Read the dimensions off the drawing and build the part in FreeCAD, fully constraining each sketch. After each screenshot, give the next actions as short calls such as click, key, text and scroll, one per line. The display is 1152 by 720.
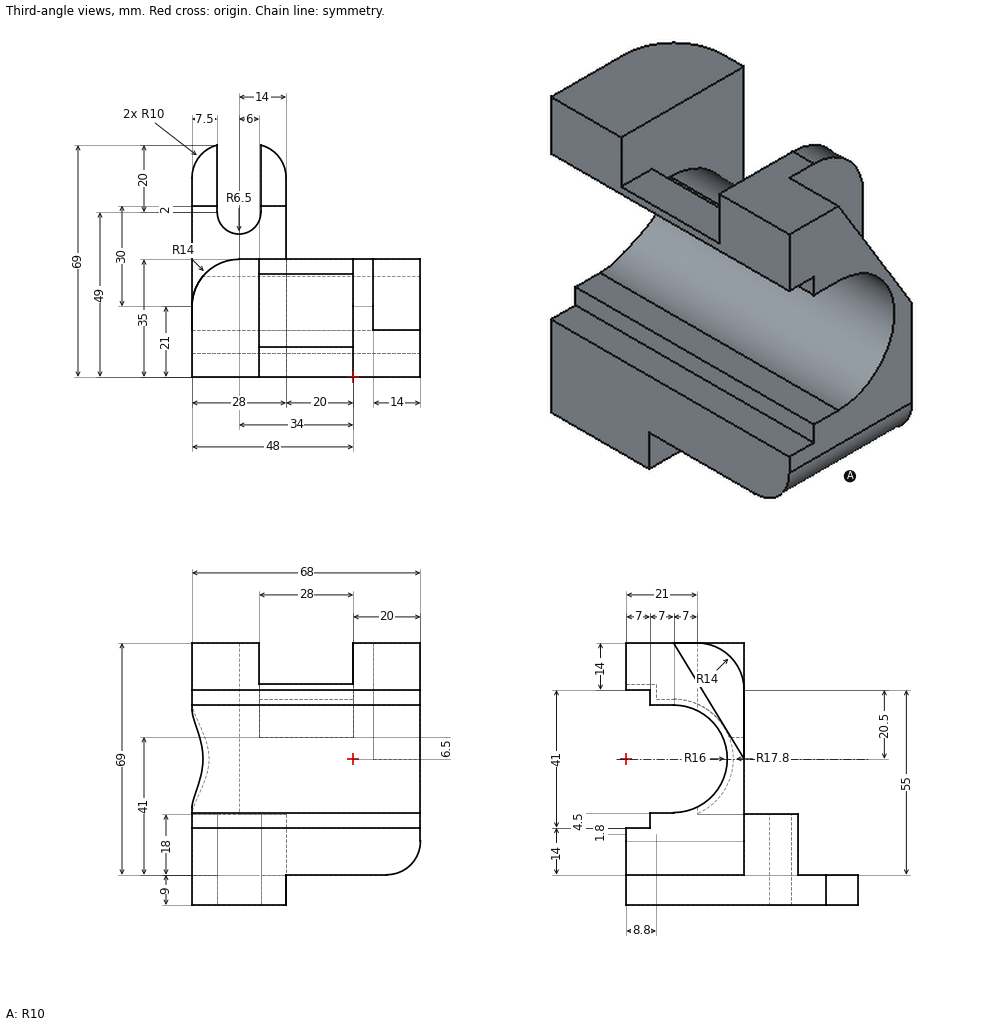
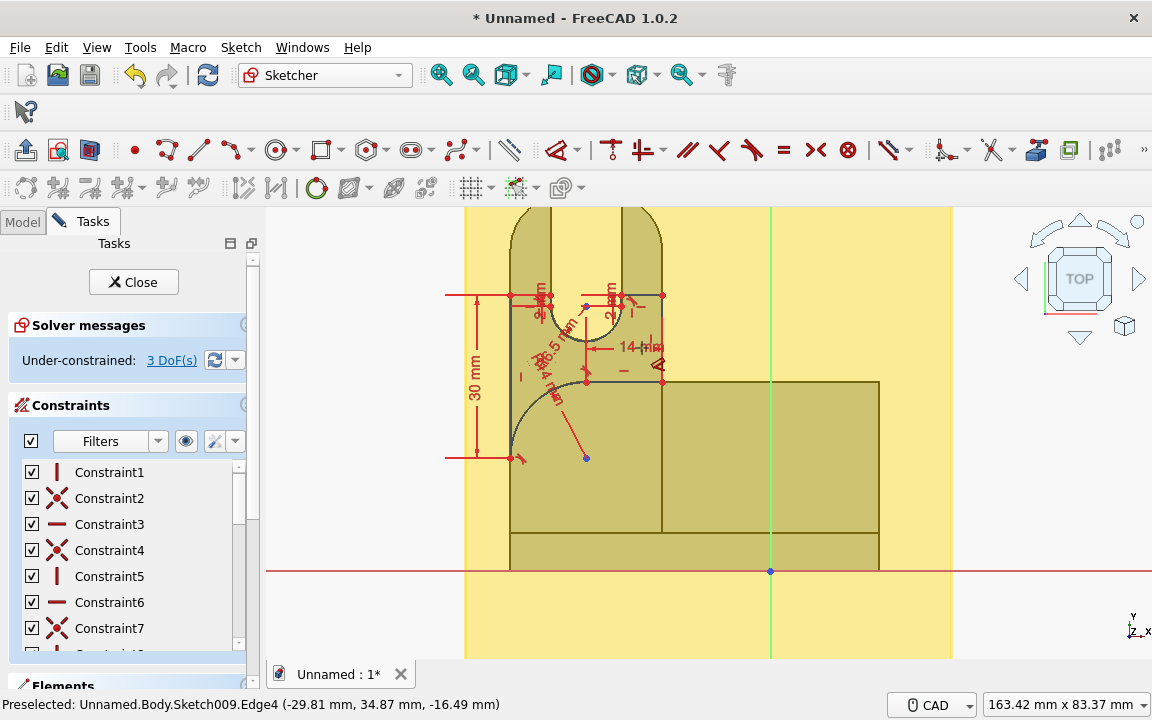
click(539, 295)
click(531, 261)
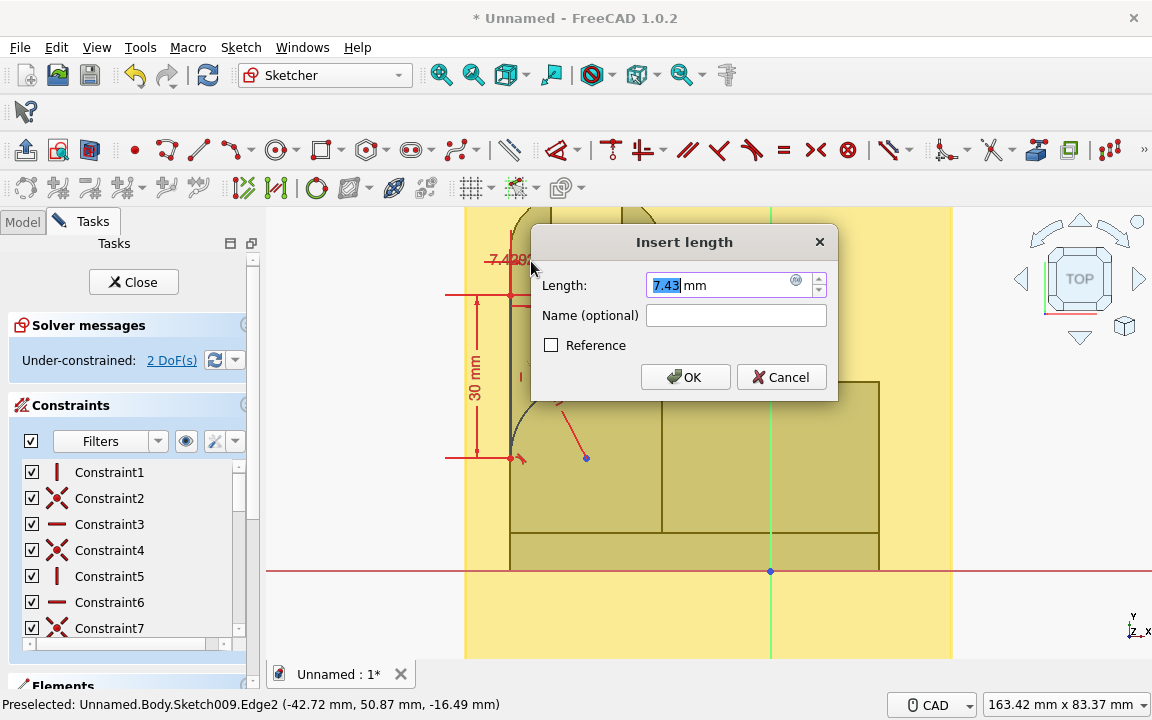
text(7.5)
key(Return)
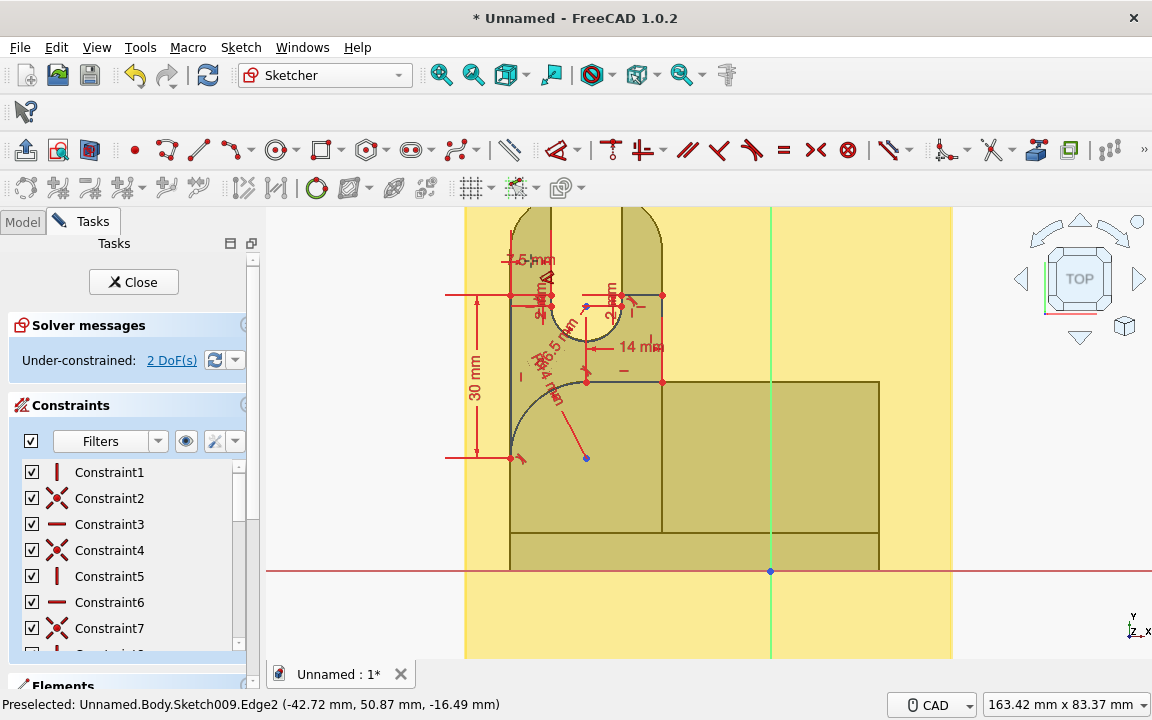
click(551, 306)
click(805, 439)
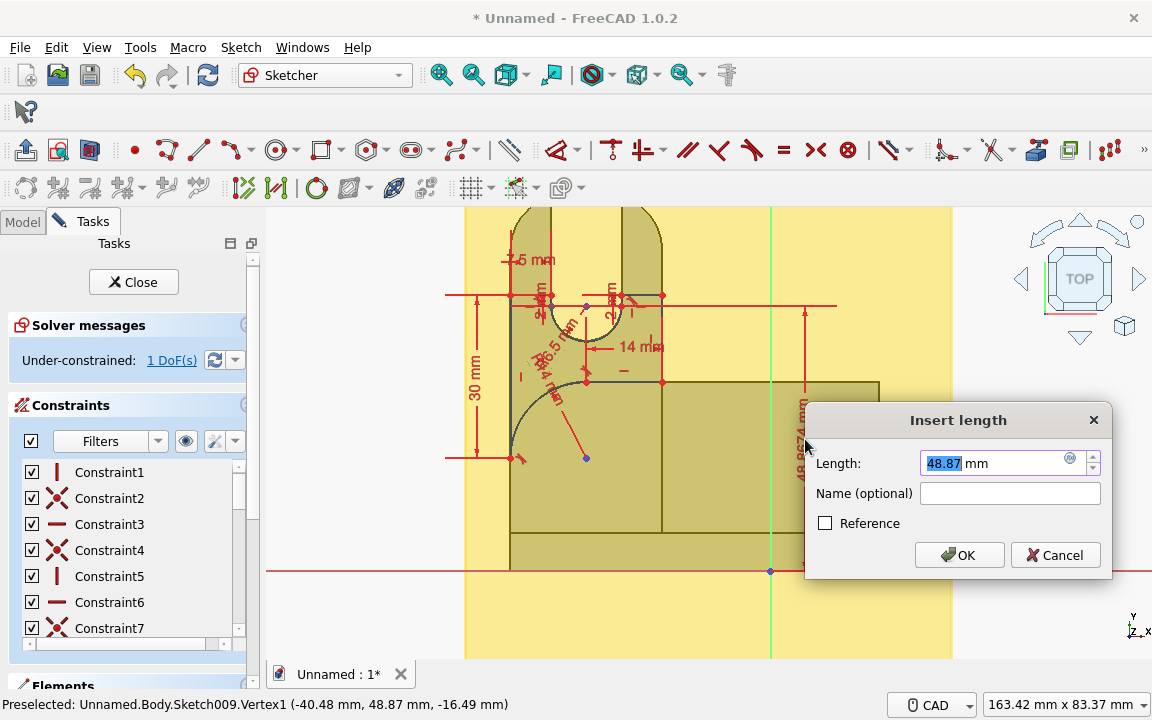
text(49)
key(Return)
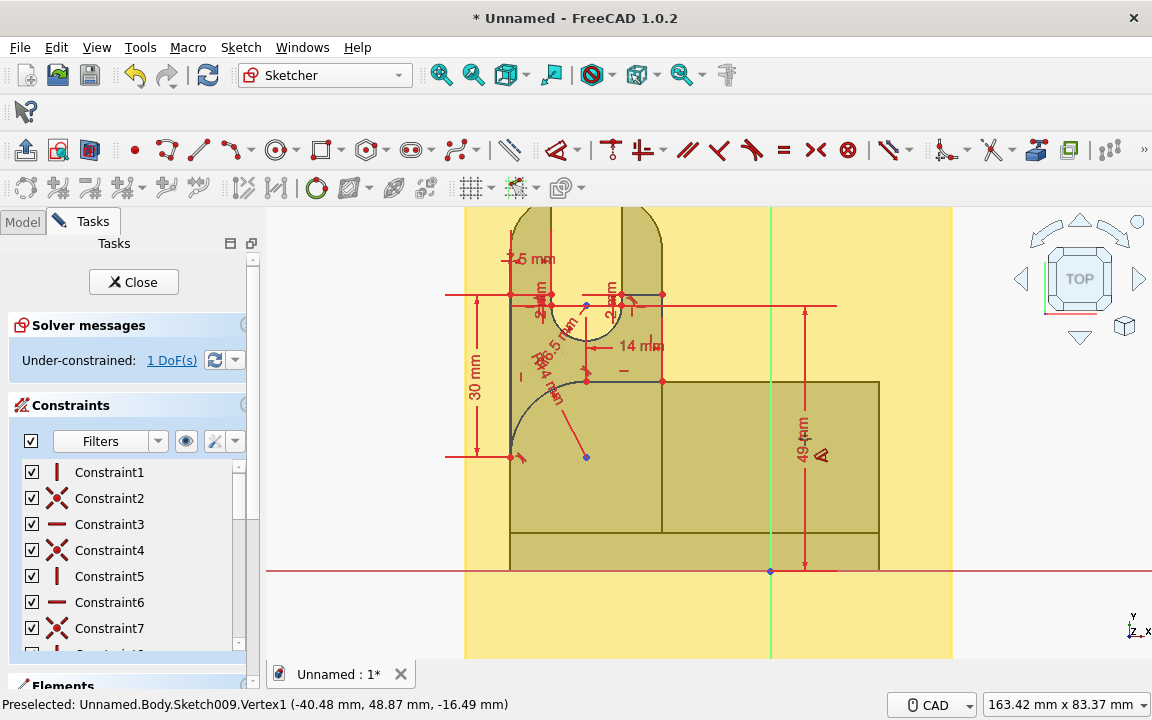
click(511, 295)
click(641, 605)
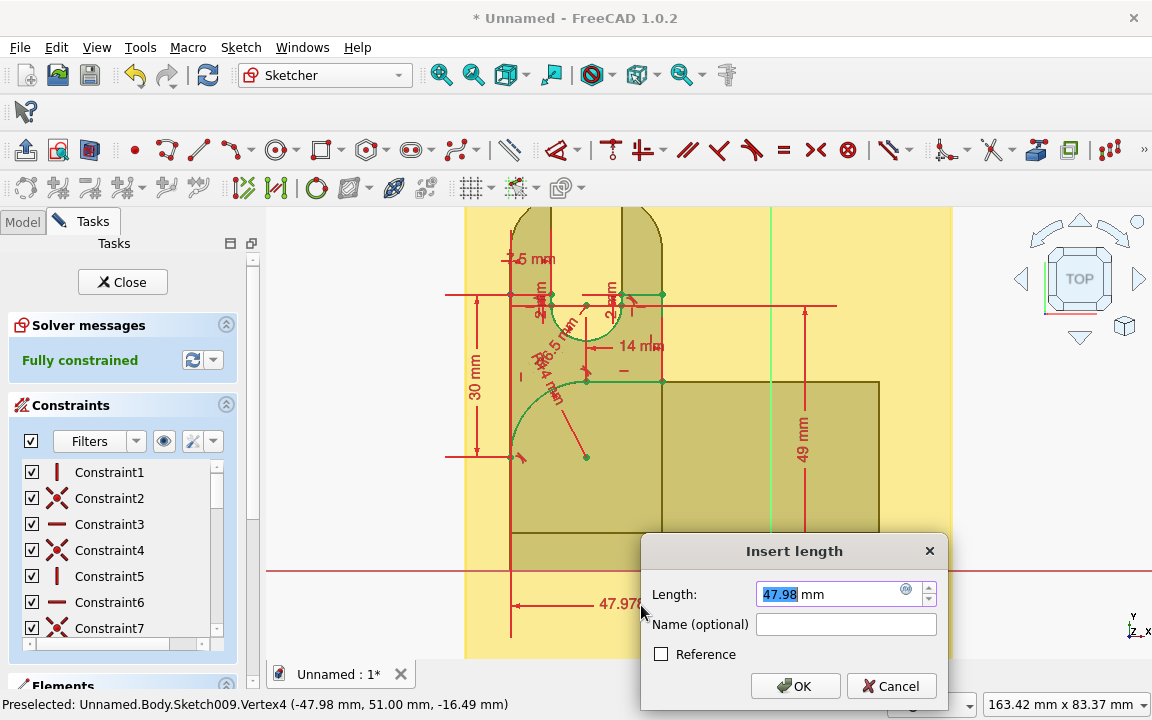
text(48)
key(Return)
key(Escape)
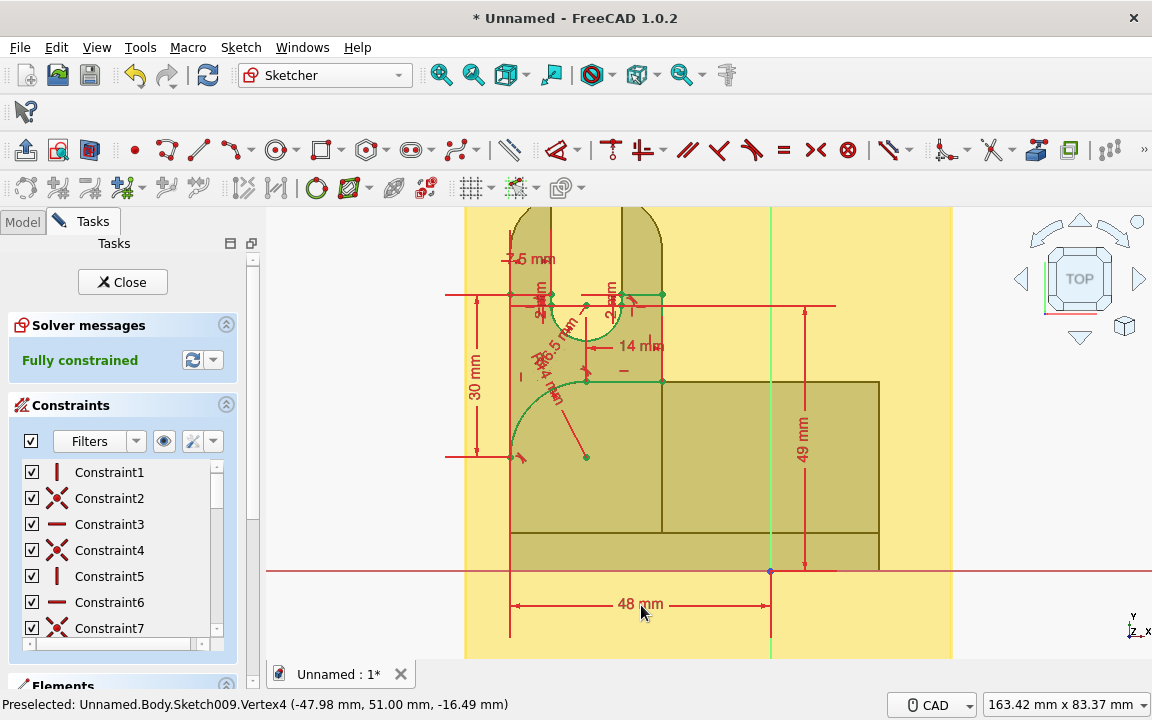
click(123, 282)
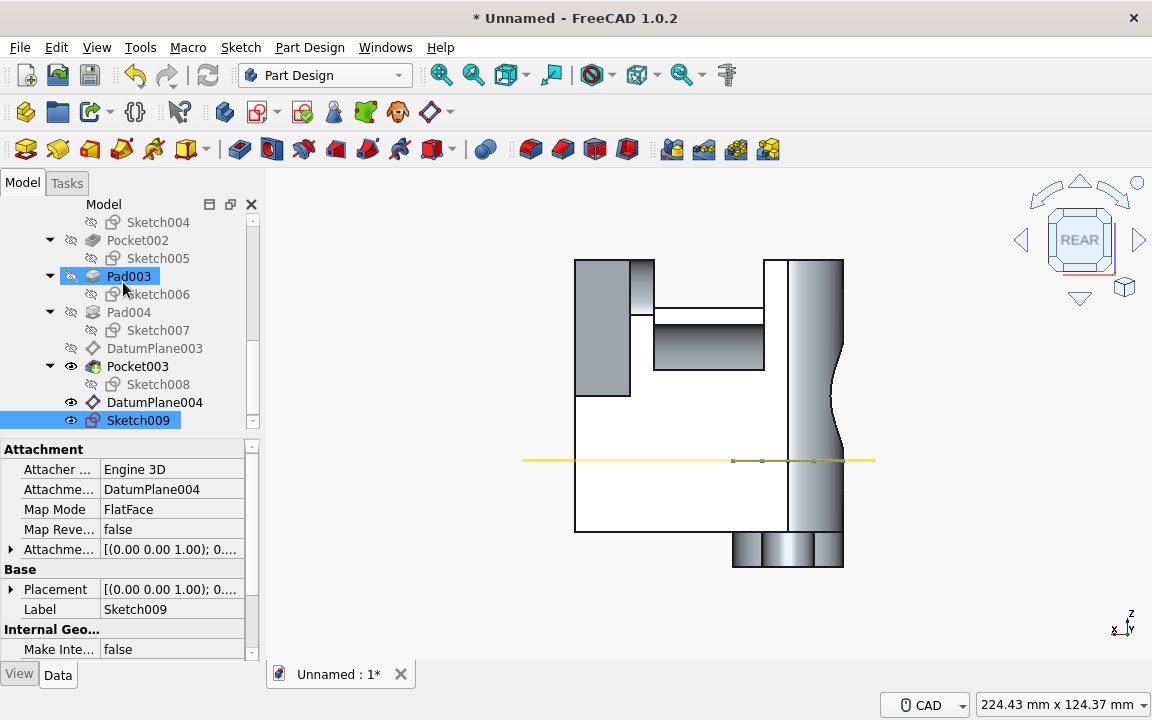
click(26, 150)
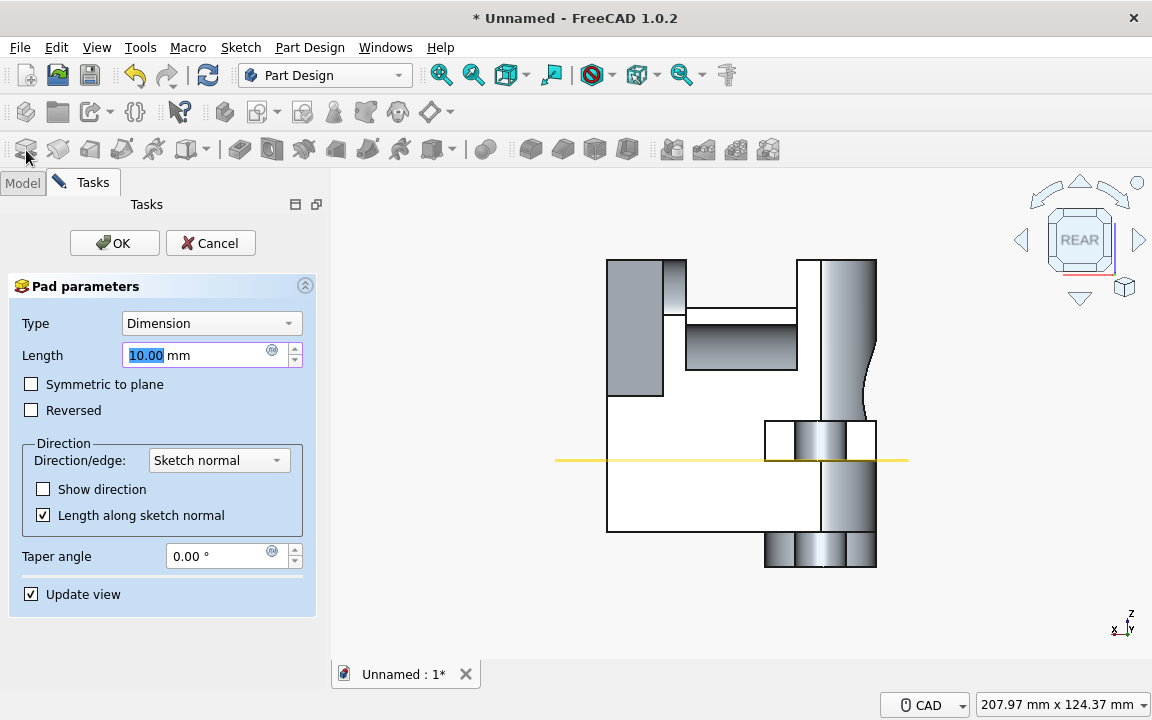
text(18)
key(Tab)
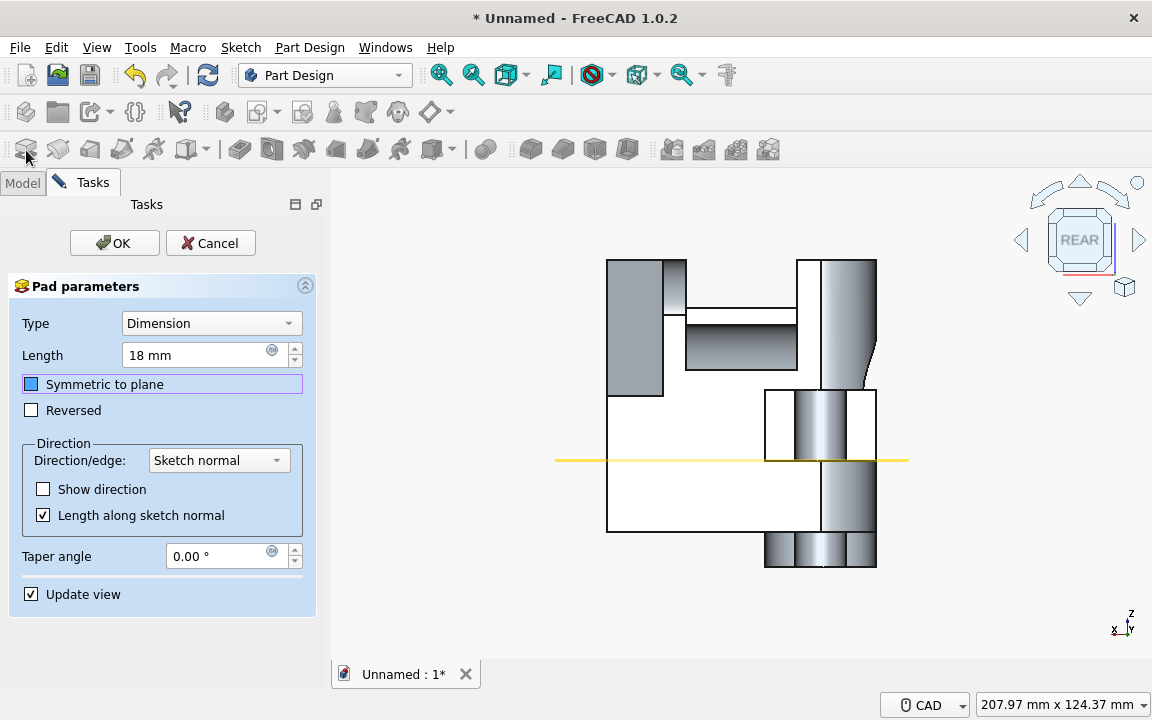
click(30, 410)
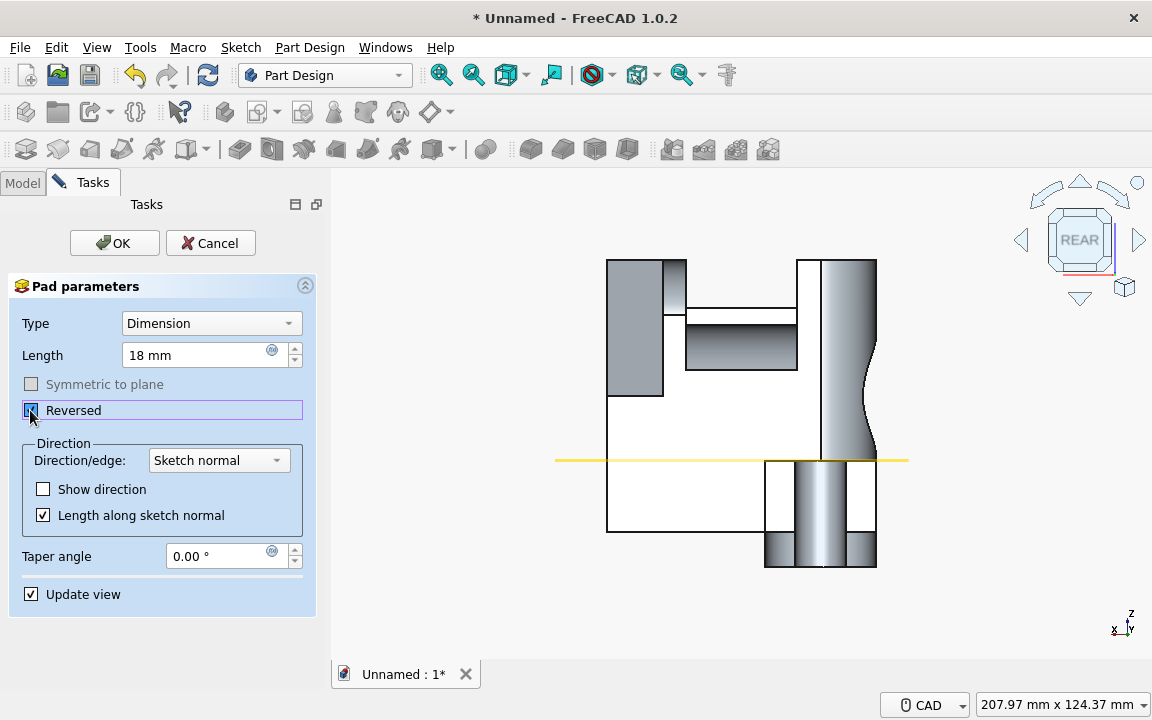
click(115, 243)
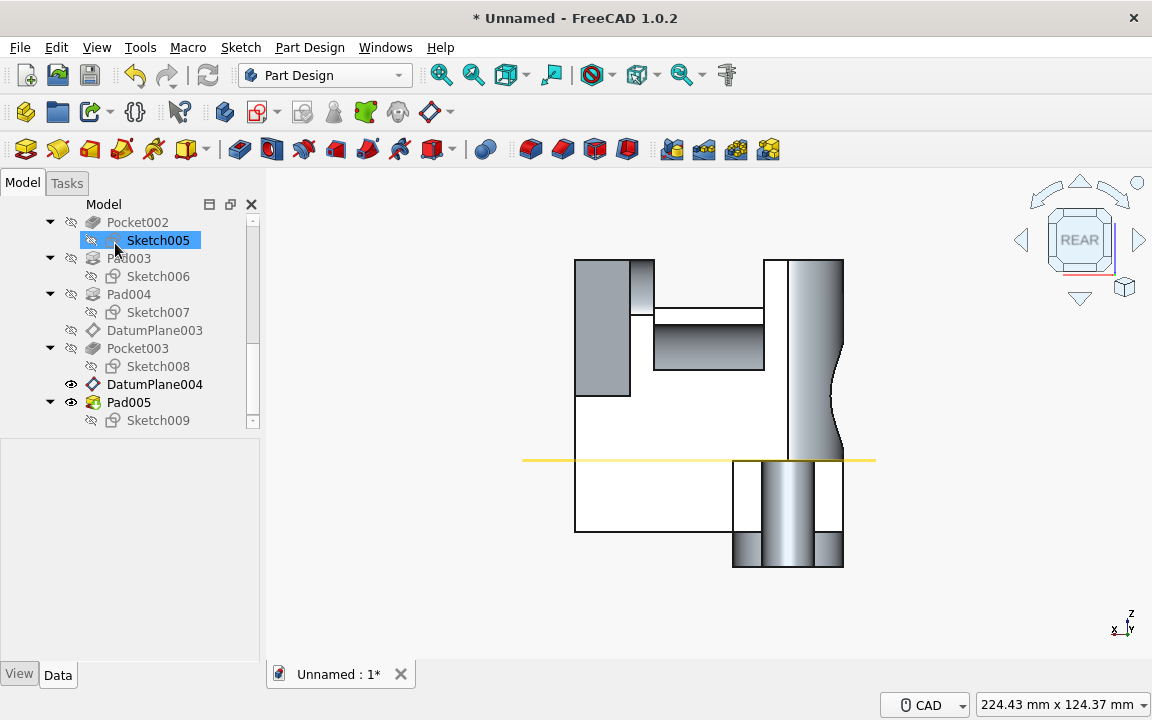
click(116, 384)
key(space)